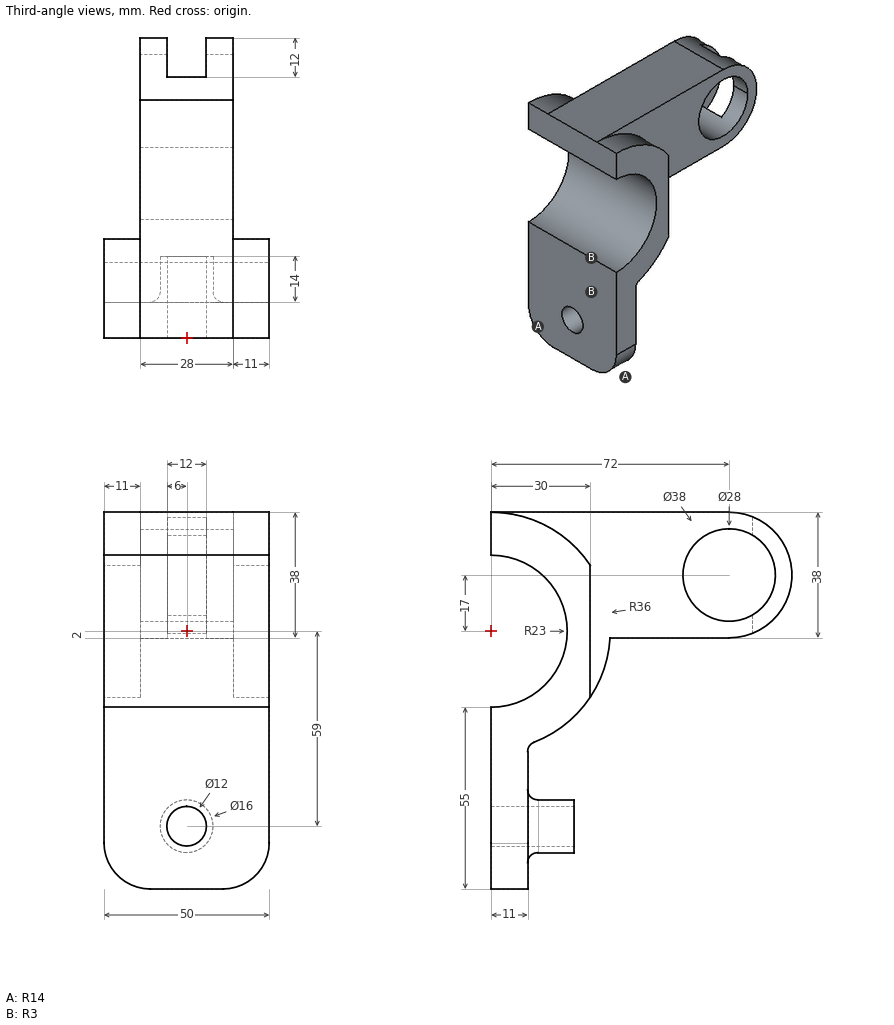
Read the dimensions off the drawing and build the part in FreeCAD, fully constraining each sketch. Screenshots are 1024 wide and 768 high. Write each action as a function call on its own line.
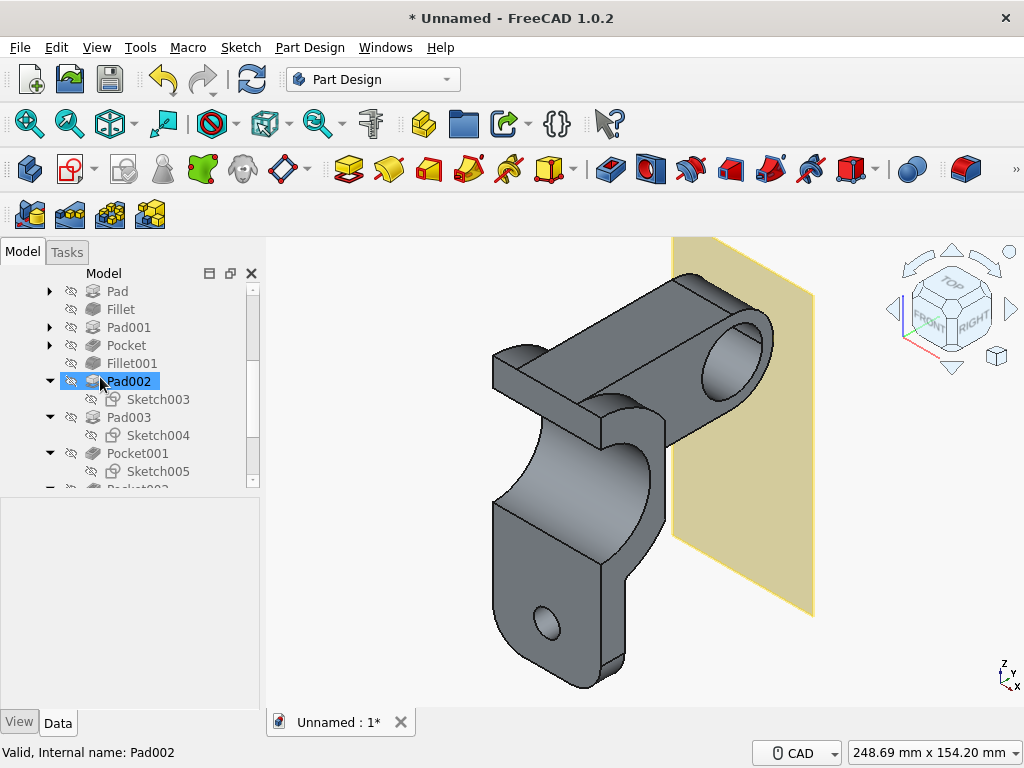
scroll(140, 377, up, 15)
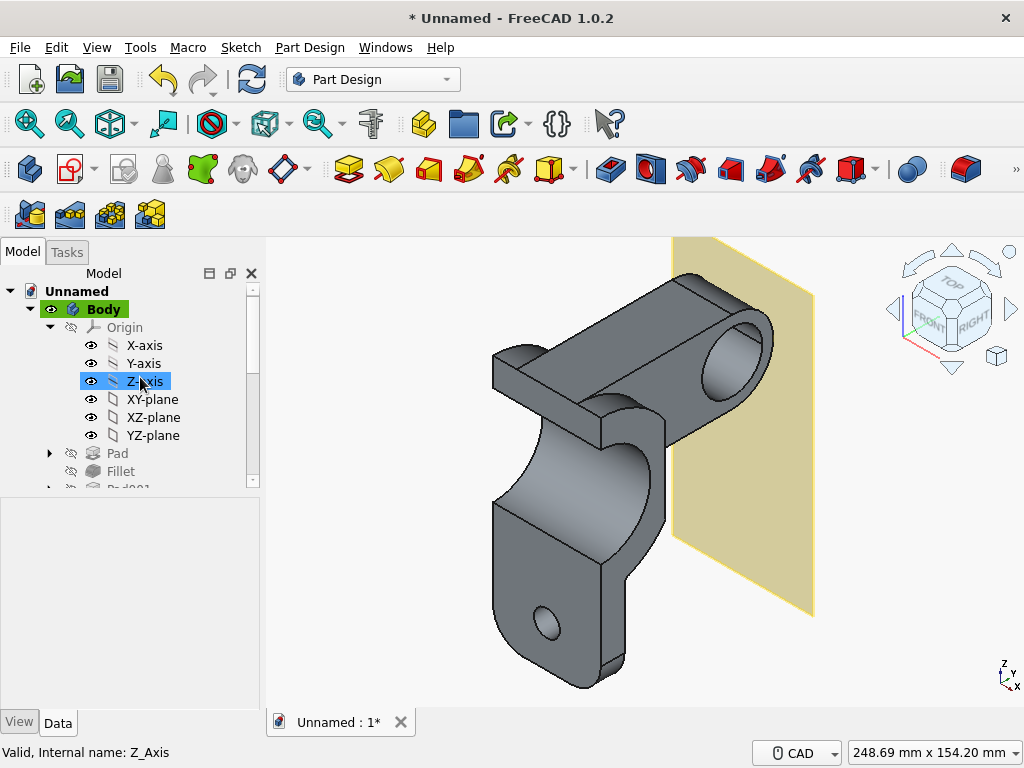
scroll(100, 377, down, 6)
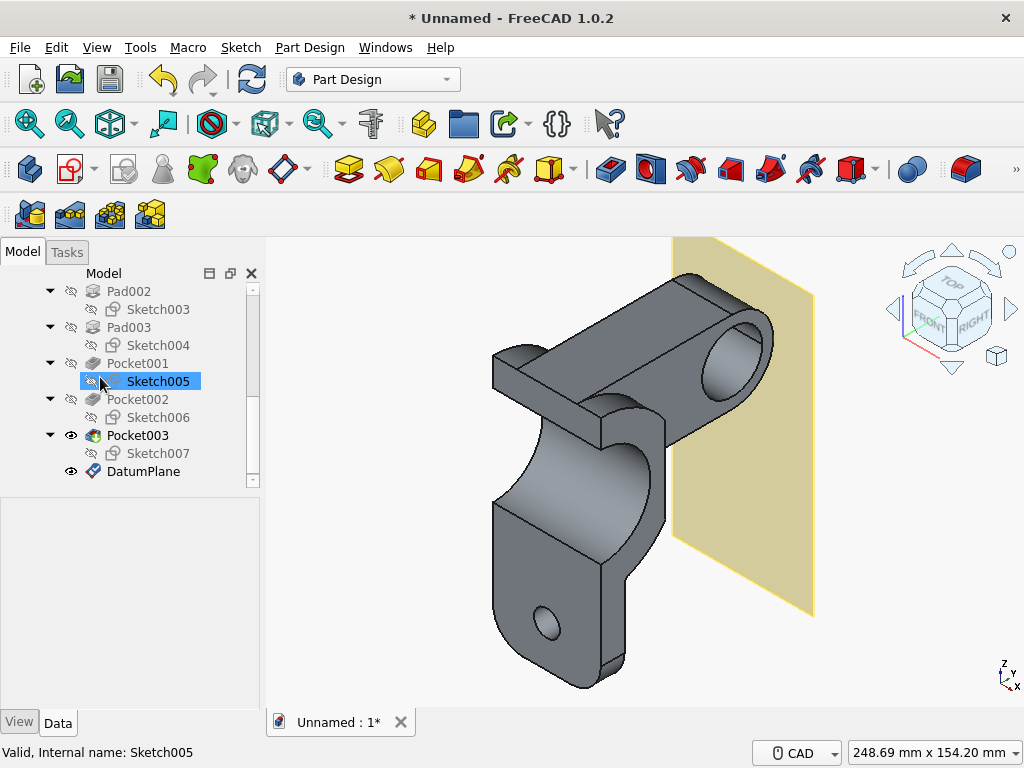
click(116, 471)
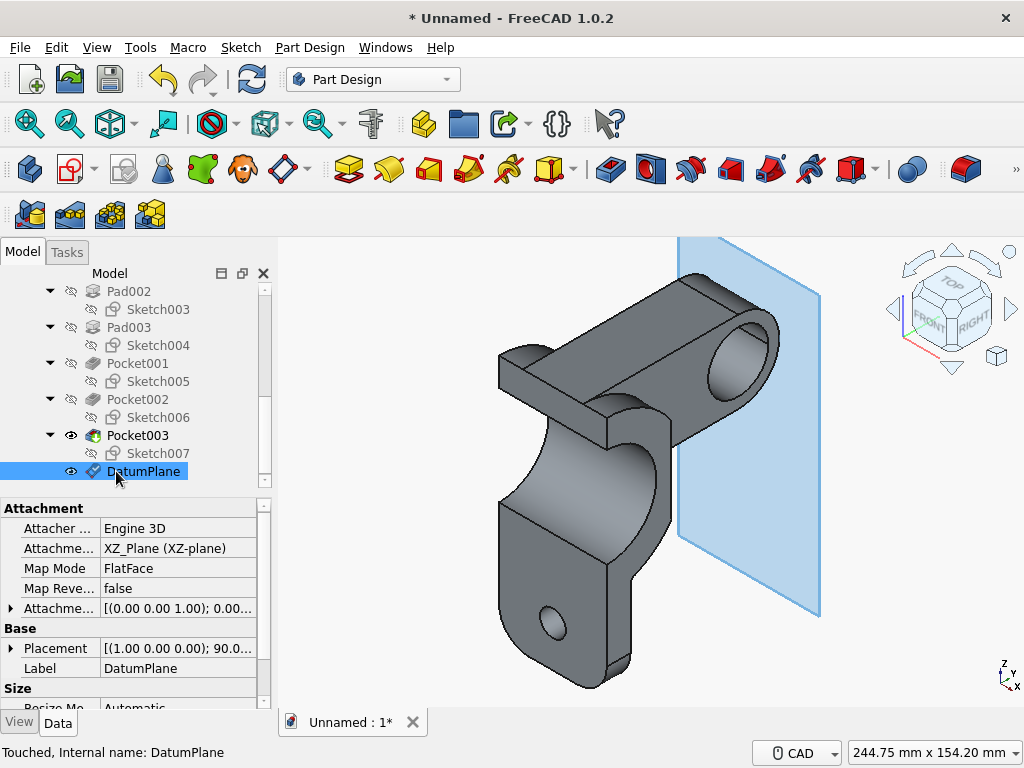
click(70, 170)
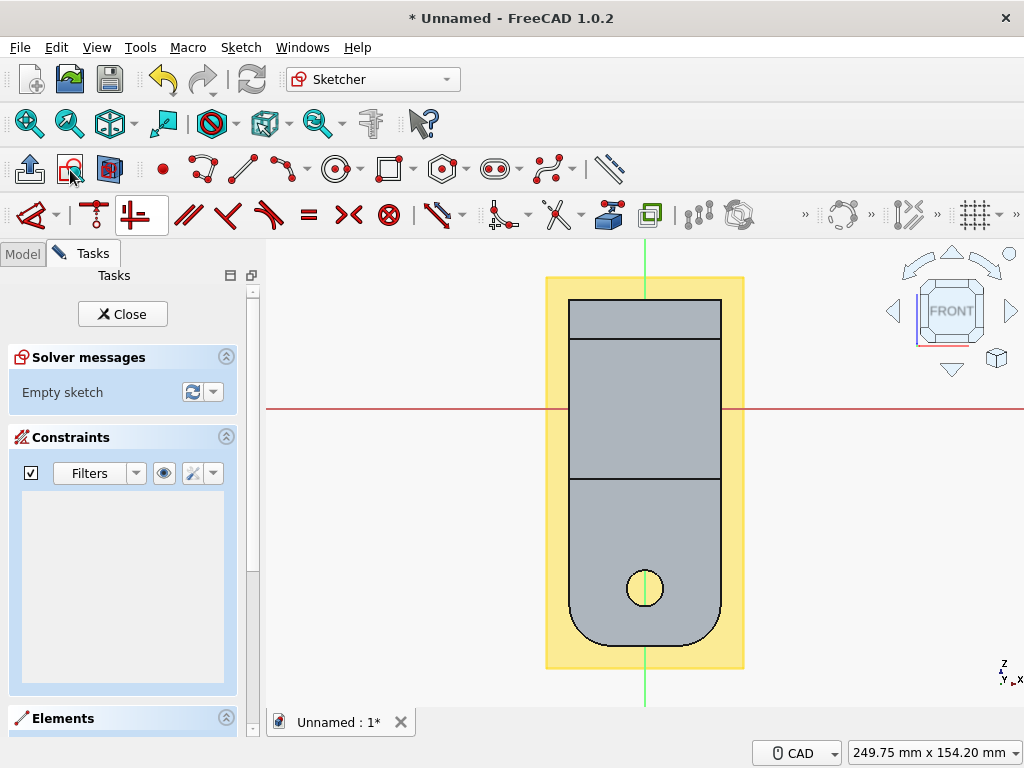
click(110, 170)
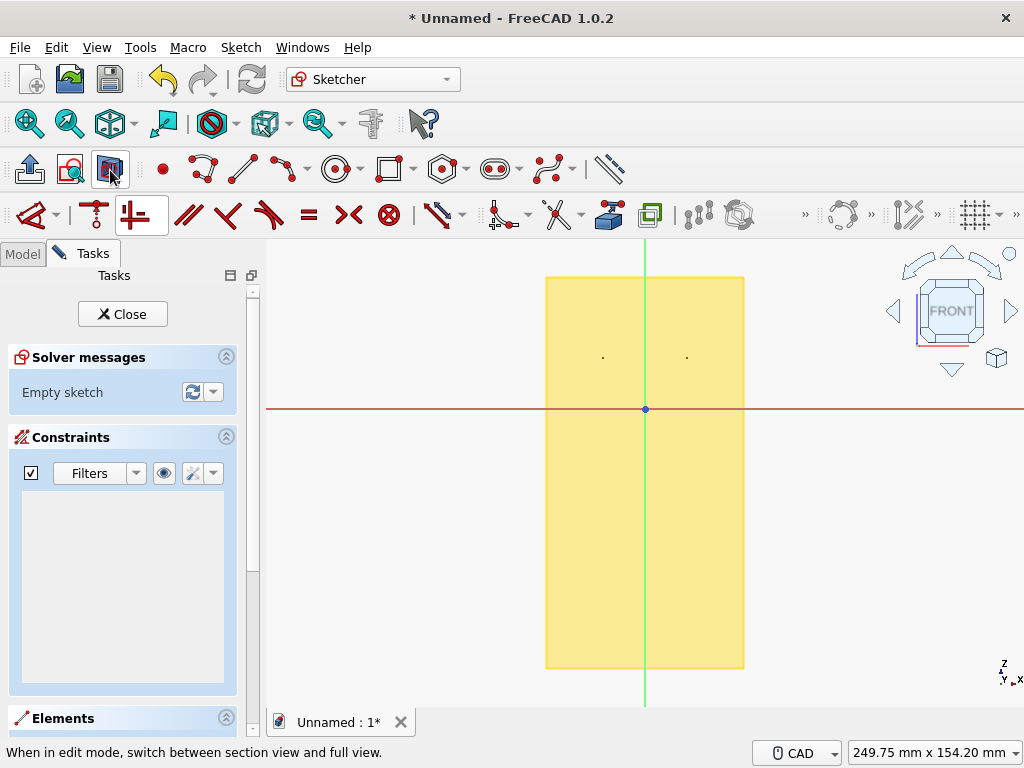
scroll(685, 291, up, 5)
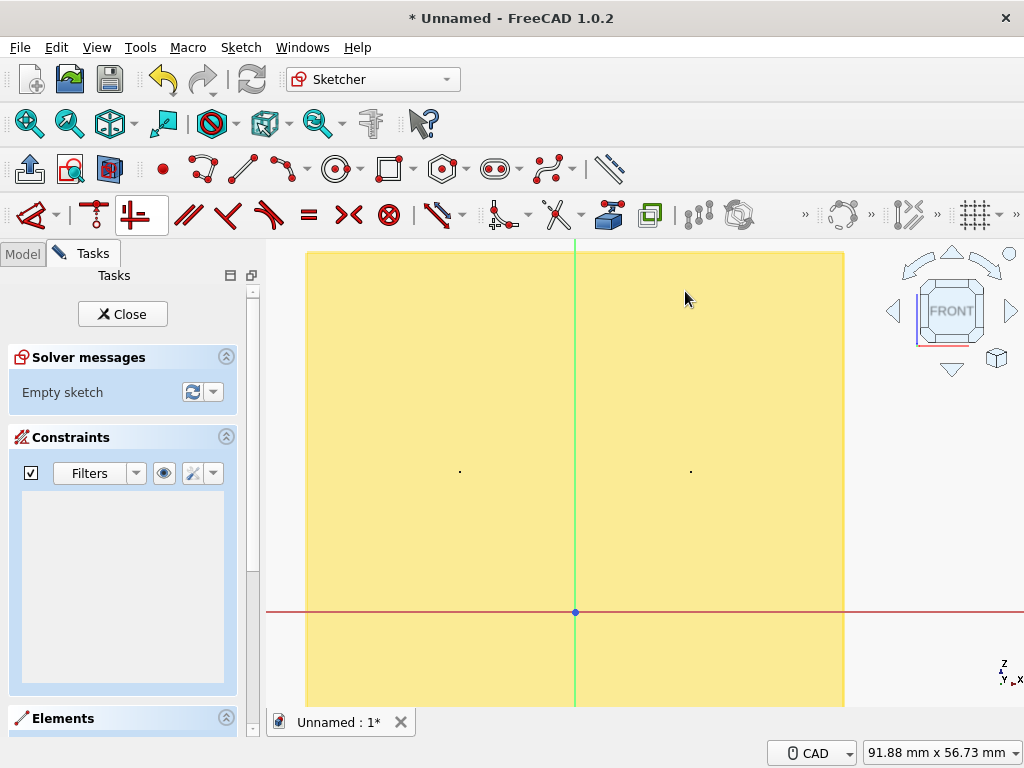
click(390, 170)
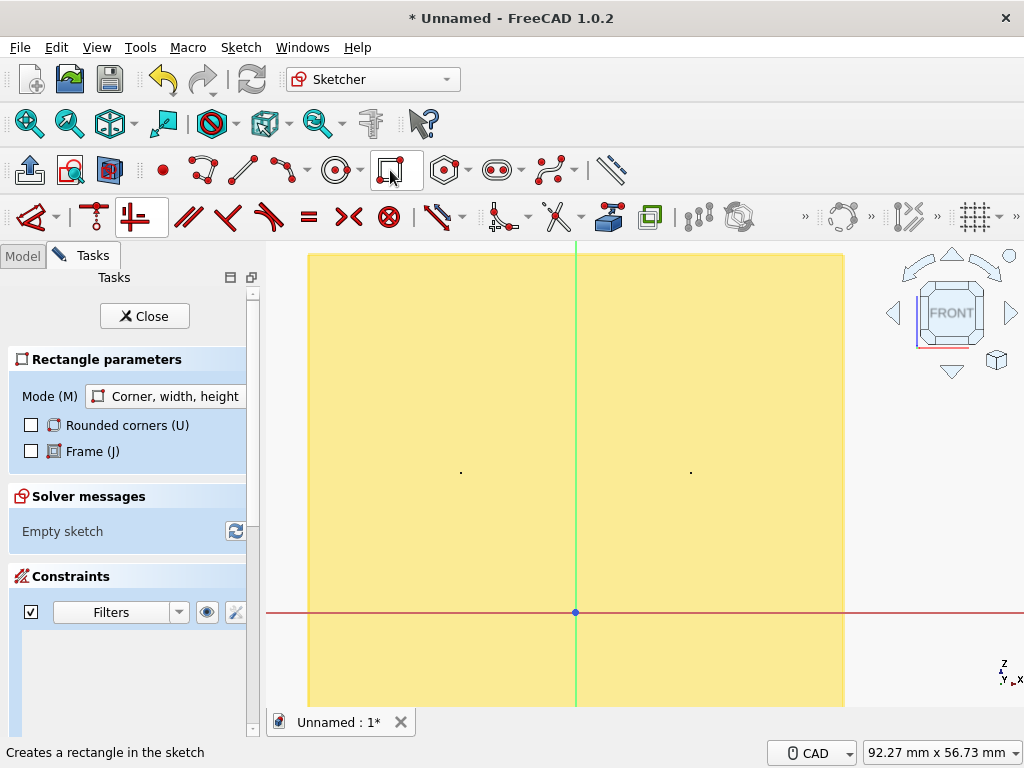
click(526, 317)
move(625, 629)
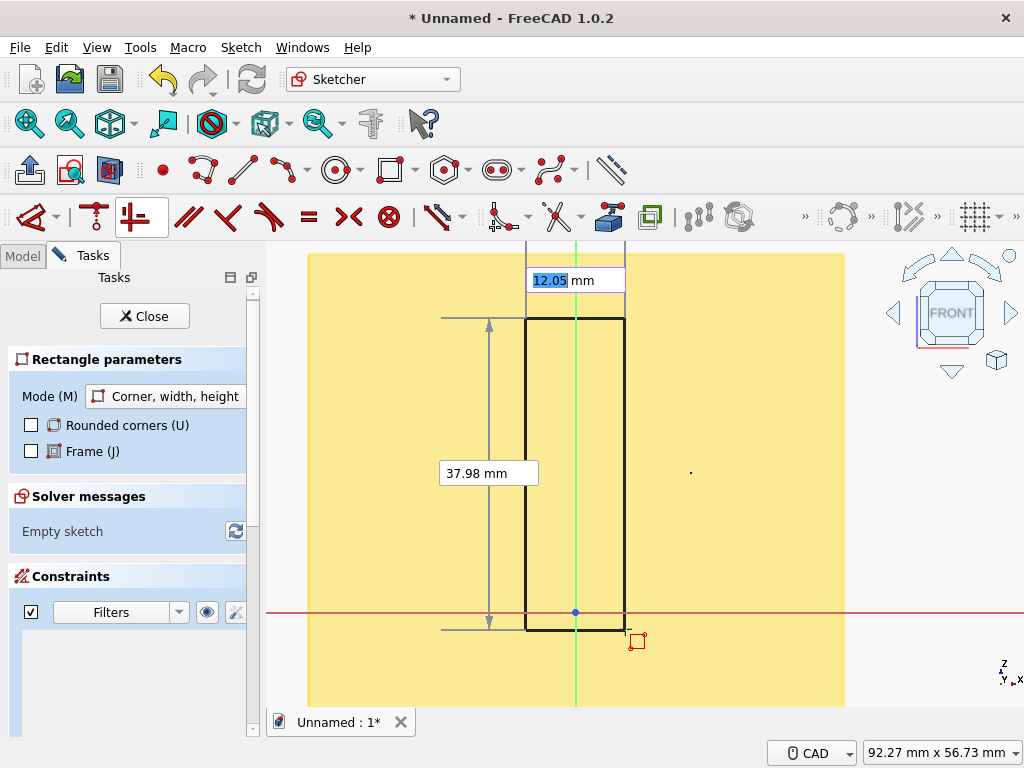
text(12)
key(Tab)
text(38)
key(Return)
key(Escape)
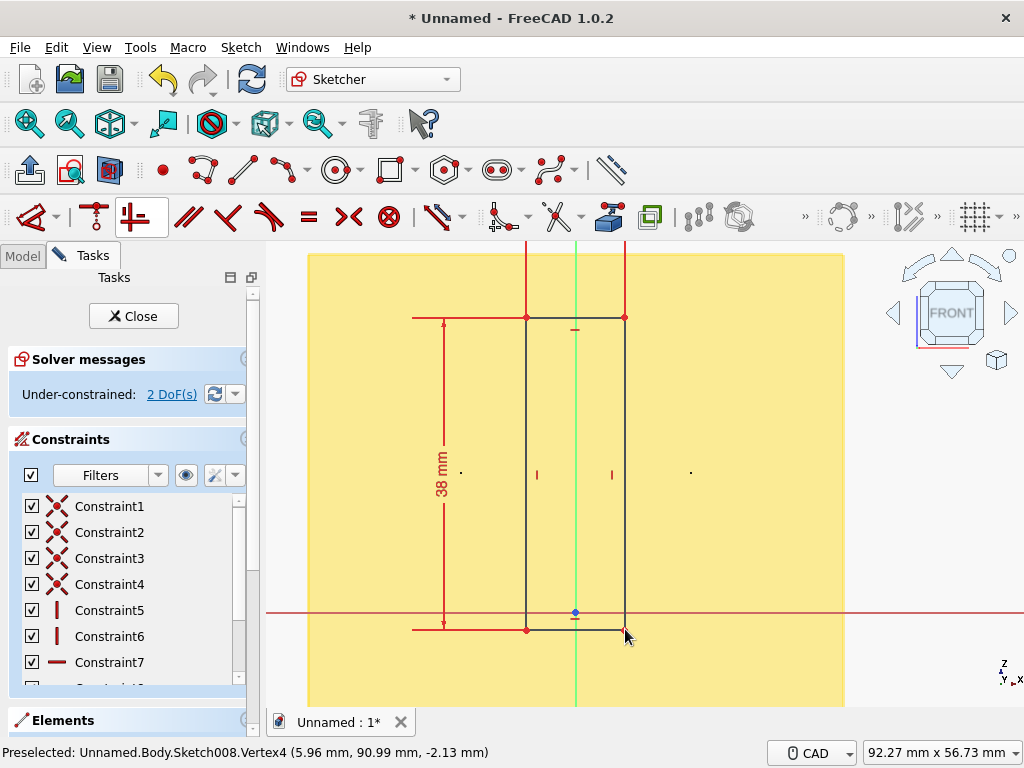
click(32, 218)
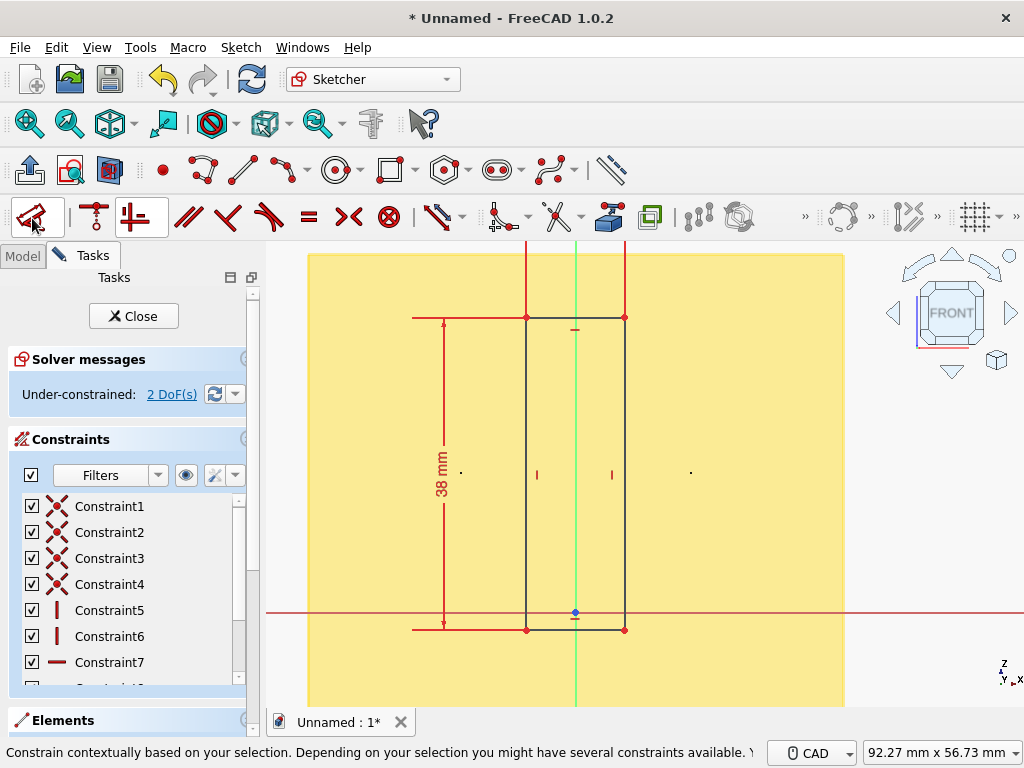
click(526, 318)
click(551, 284)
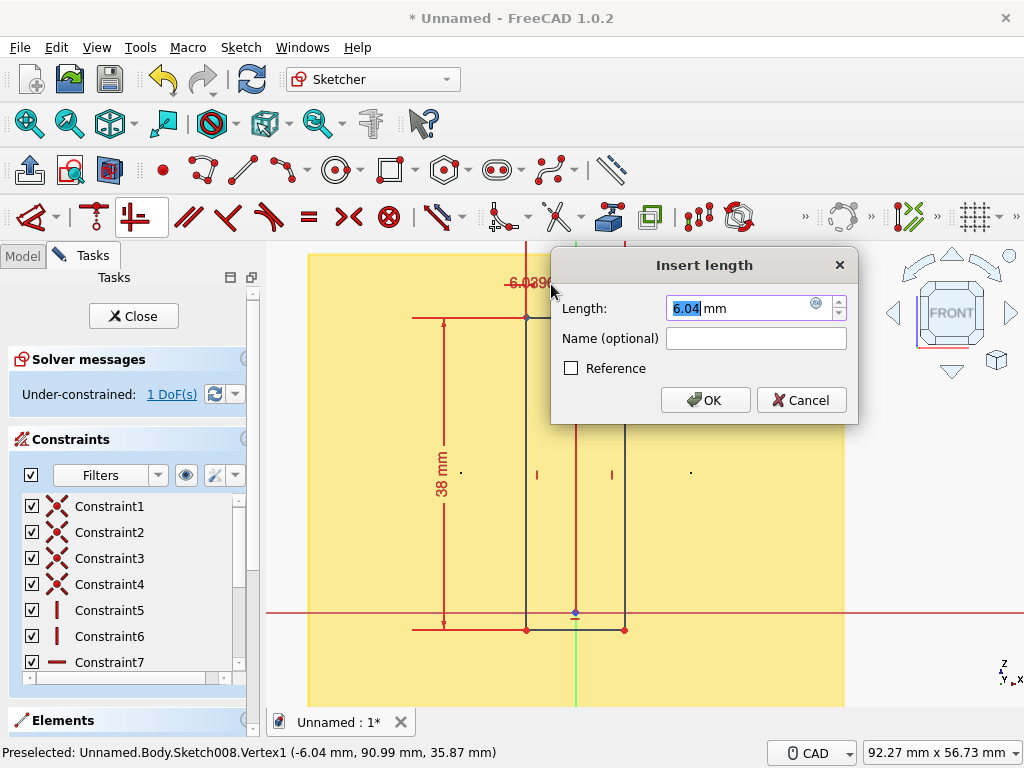
text(6)
key(Return)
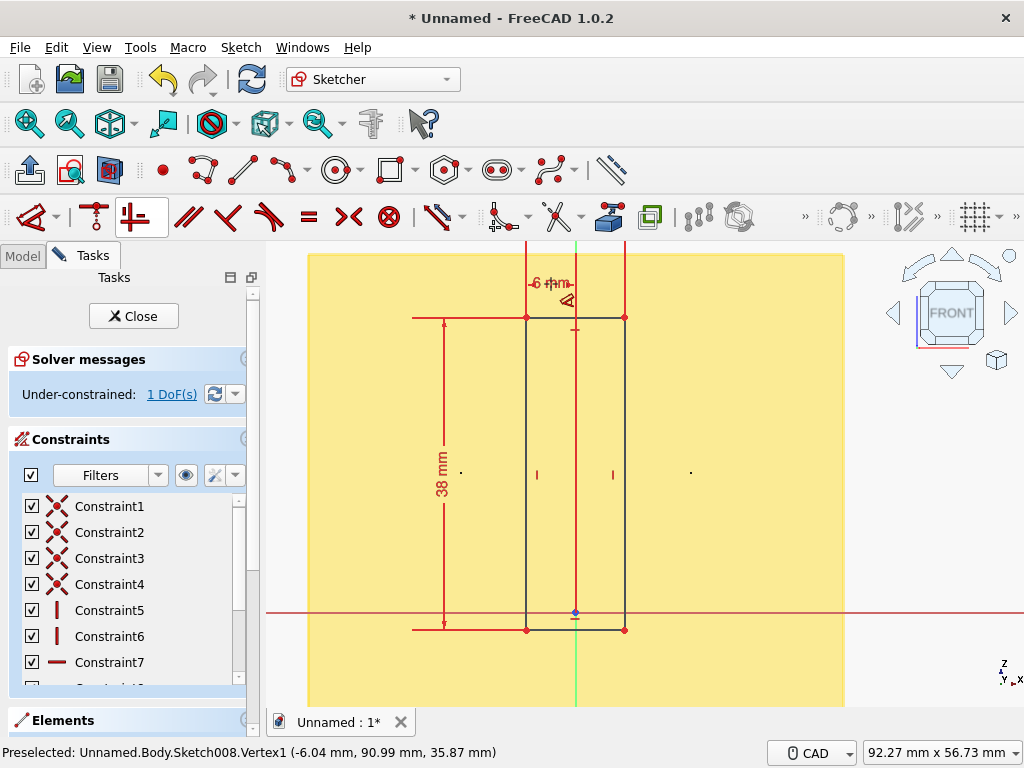
scroll(526, 630, up, 5)